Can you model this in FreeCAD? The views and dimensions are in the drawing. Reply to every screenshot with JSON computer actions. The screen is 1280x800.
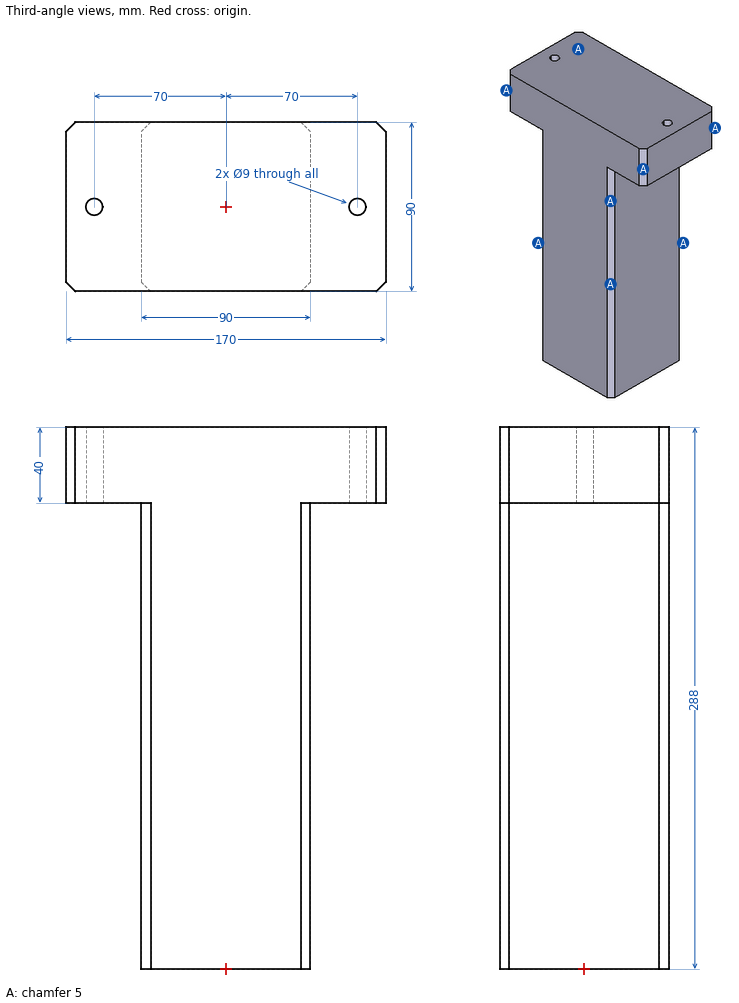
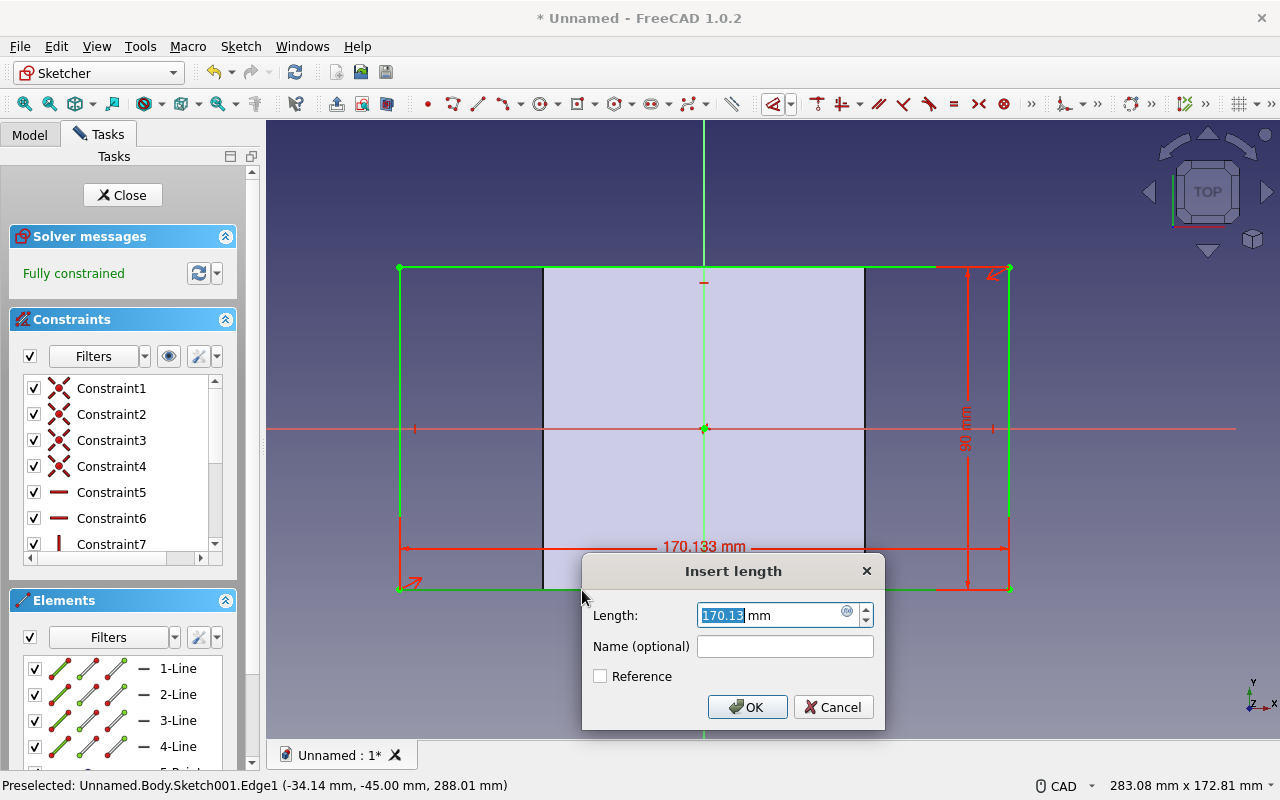
{"action": "type", "text": "170"}
{"action": "key", "text": "Return"}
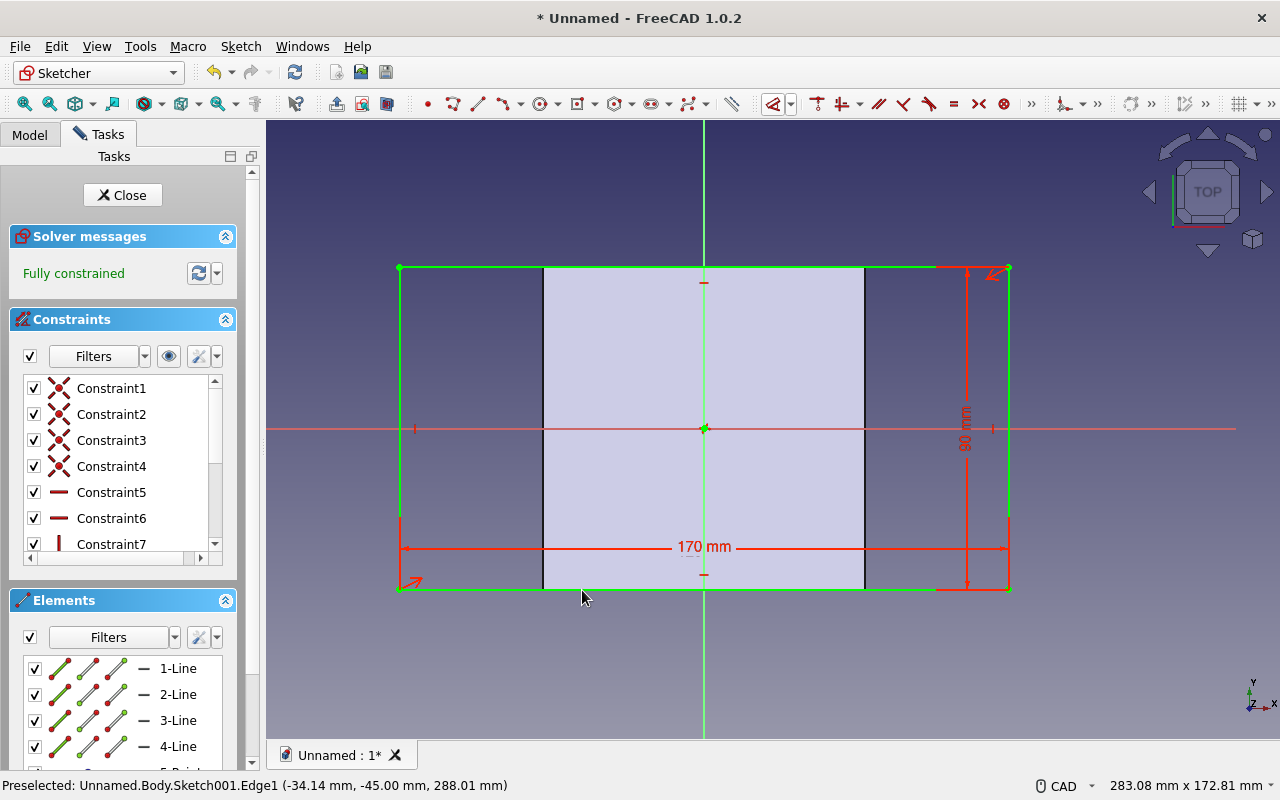
{"action": "left_click", "coordinate": [123, 195]}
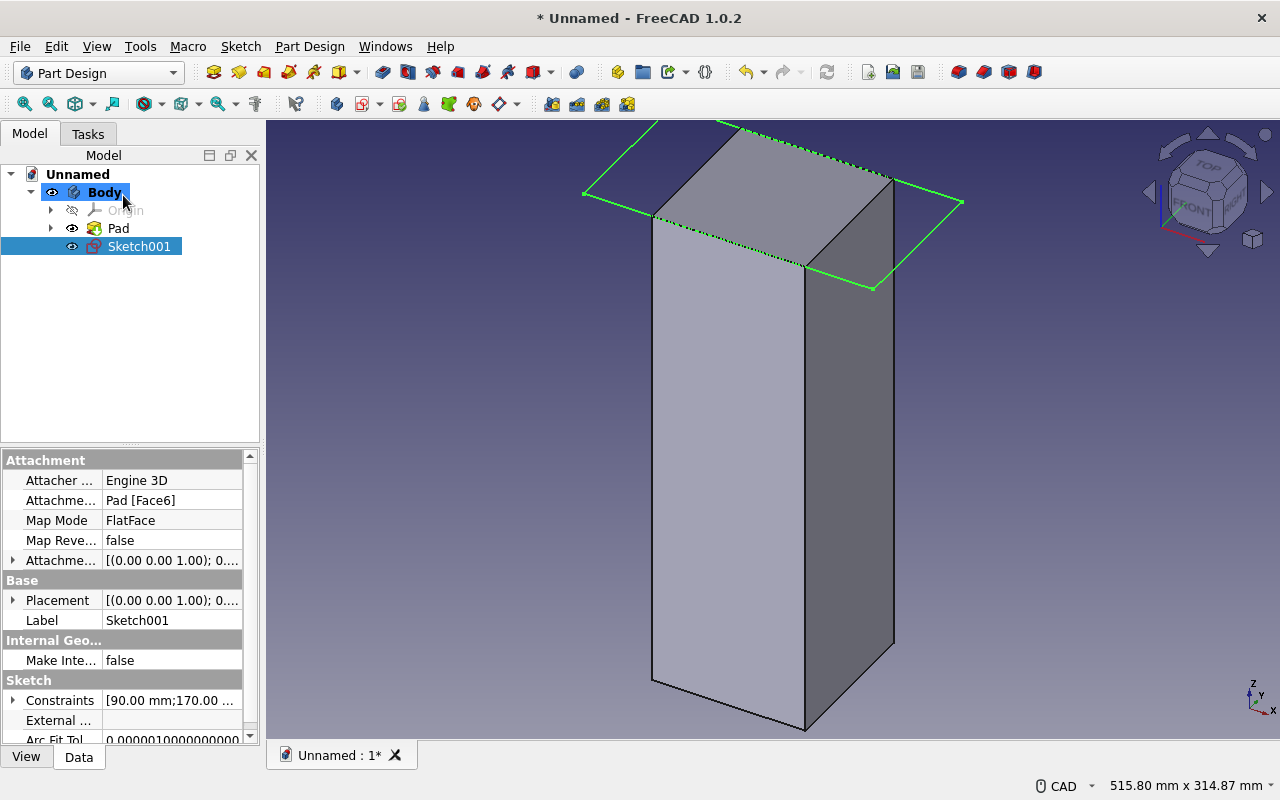
{"action": "left_click", "coordinate": [214, 72]}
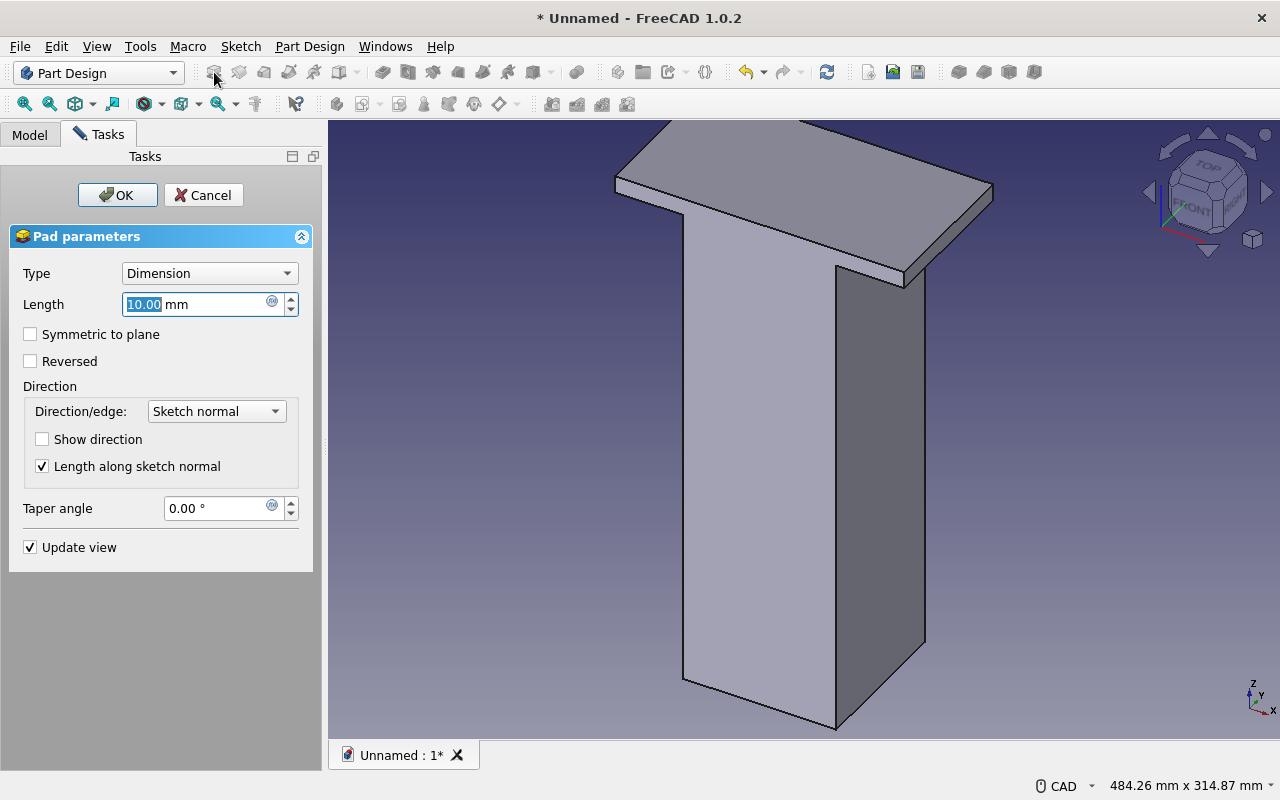
{"action": "type", "text": "40"}
{"action": "key", "text": "Tab"}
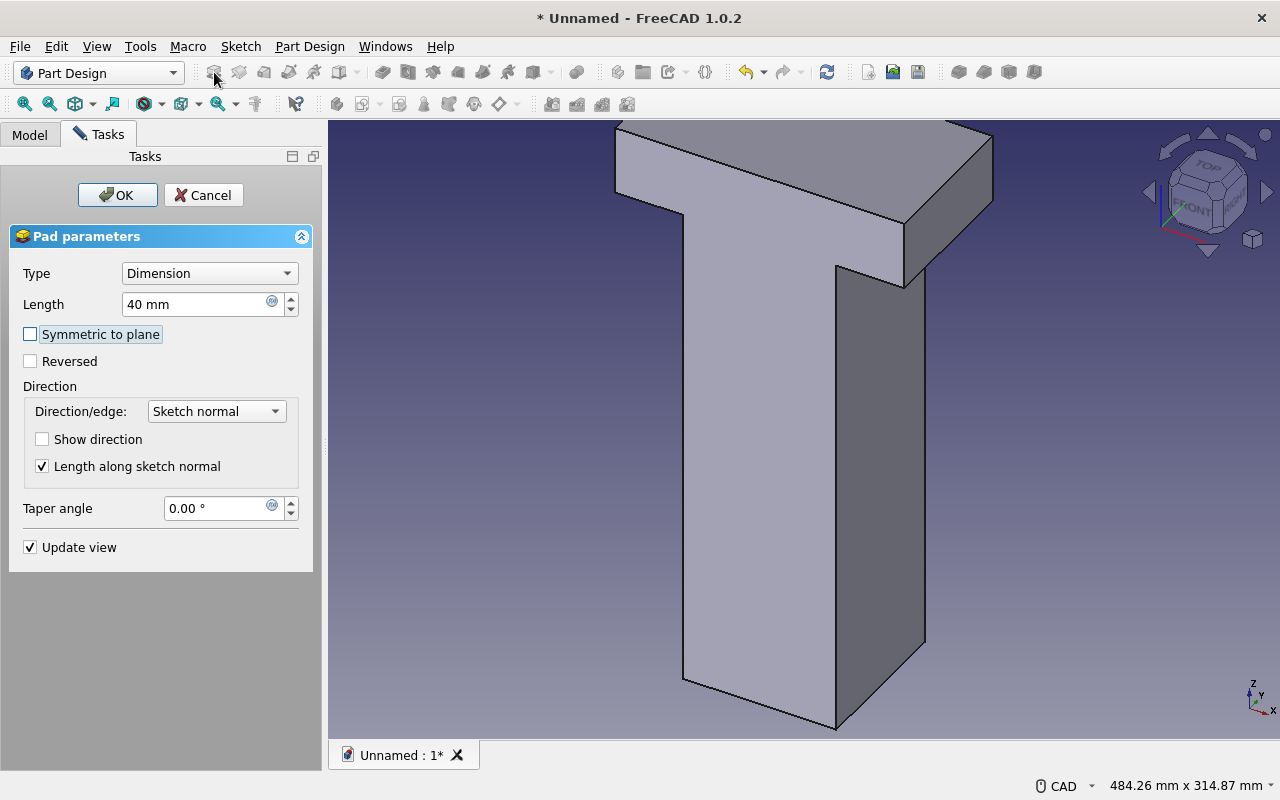
{"action": "left_click", "coordinate": [31, 361]}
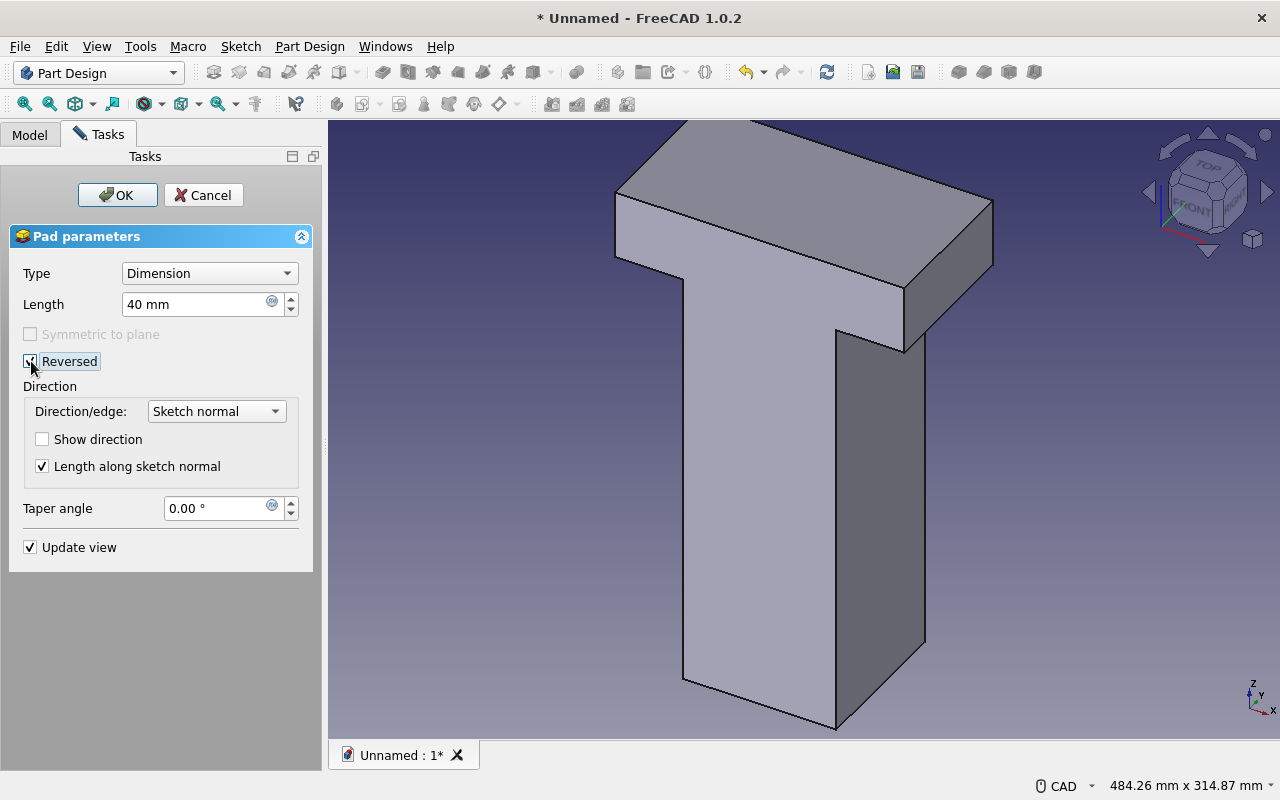
{"action": "left_click", "coordinate": [118, 195]}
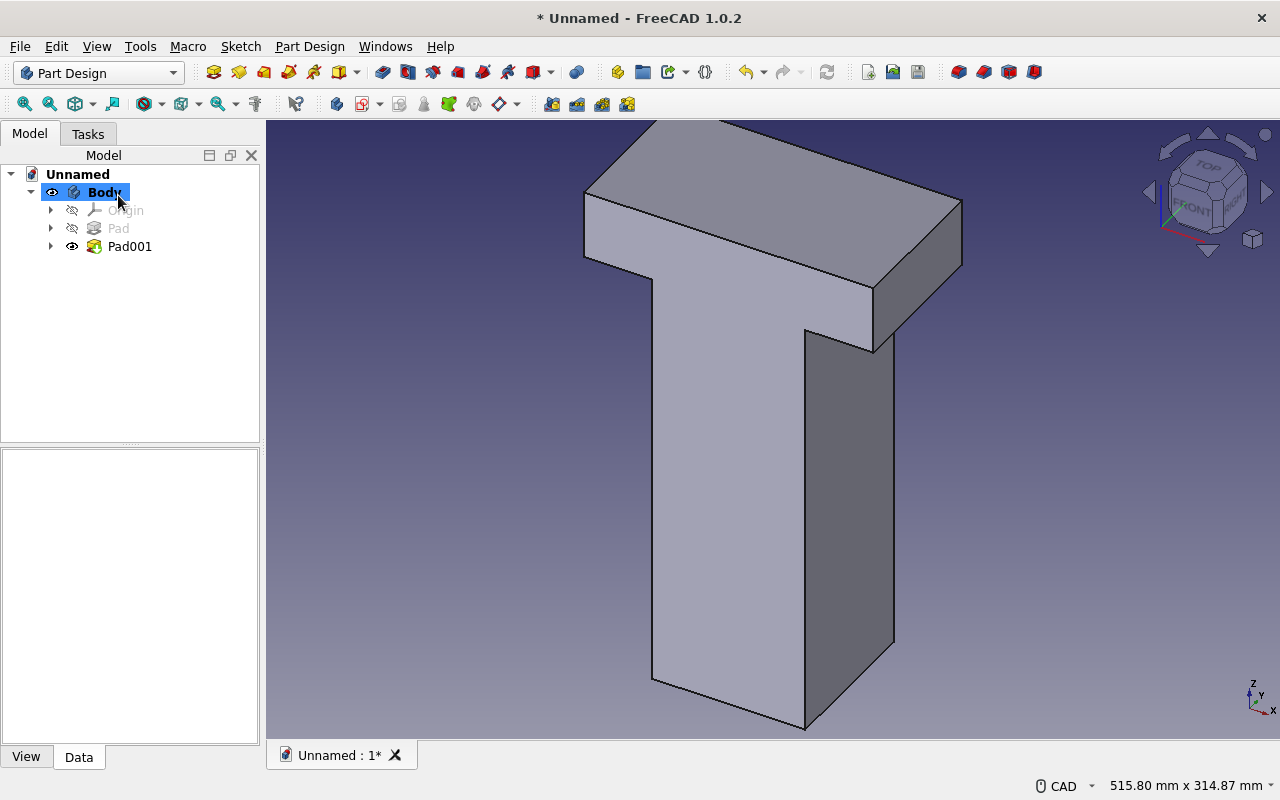
{"action": "left_click", "coordinate": [25, 104]}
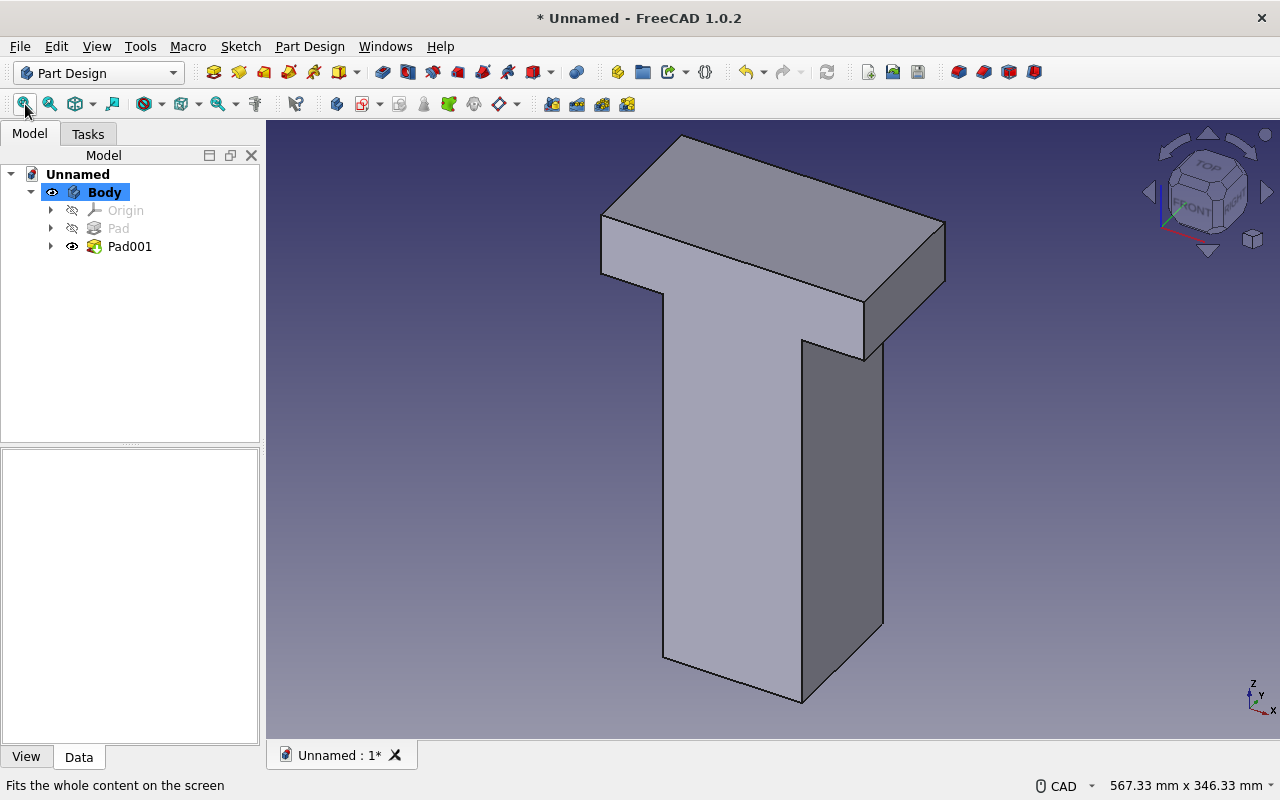
{"action": "left_click", "coordinate": [802, 521]}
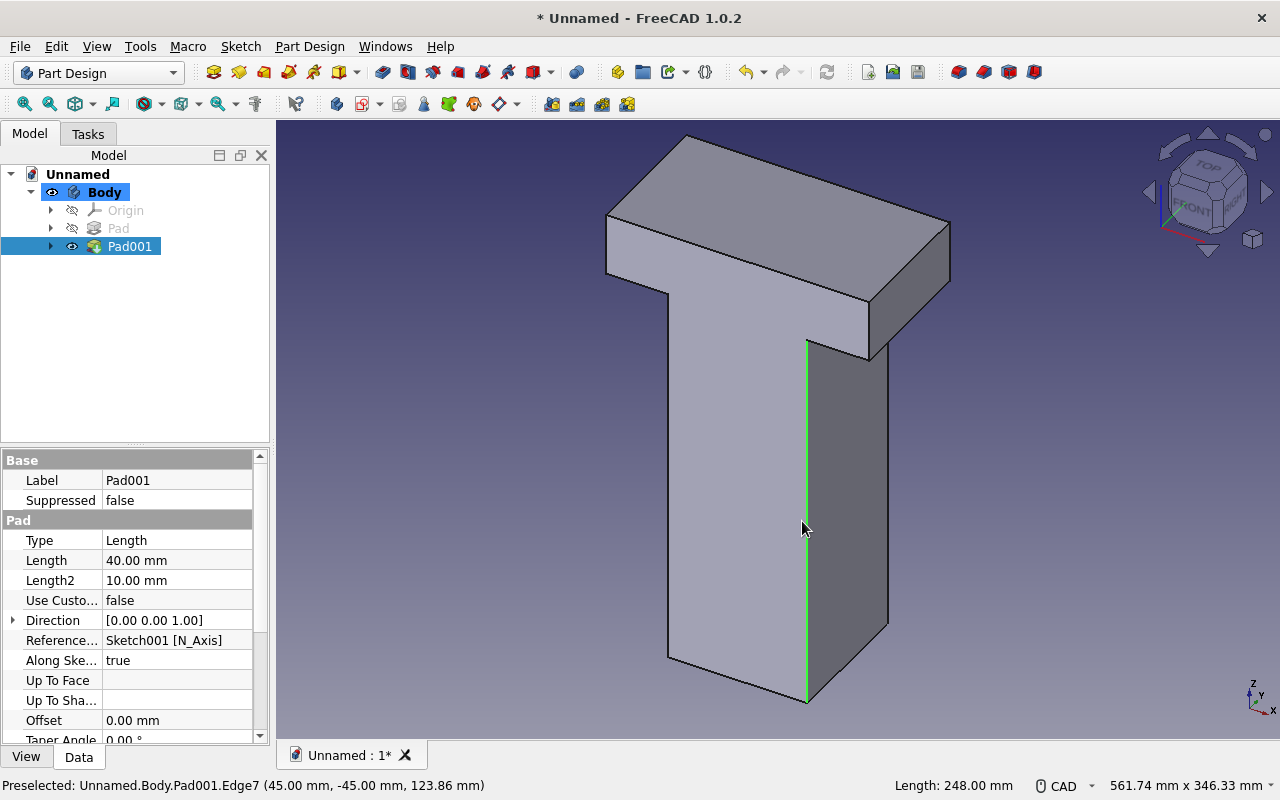
{"action": "left_click", "coordinate": [869, 330], "text": "ctrl"}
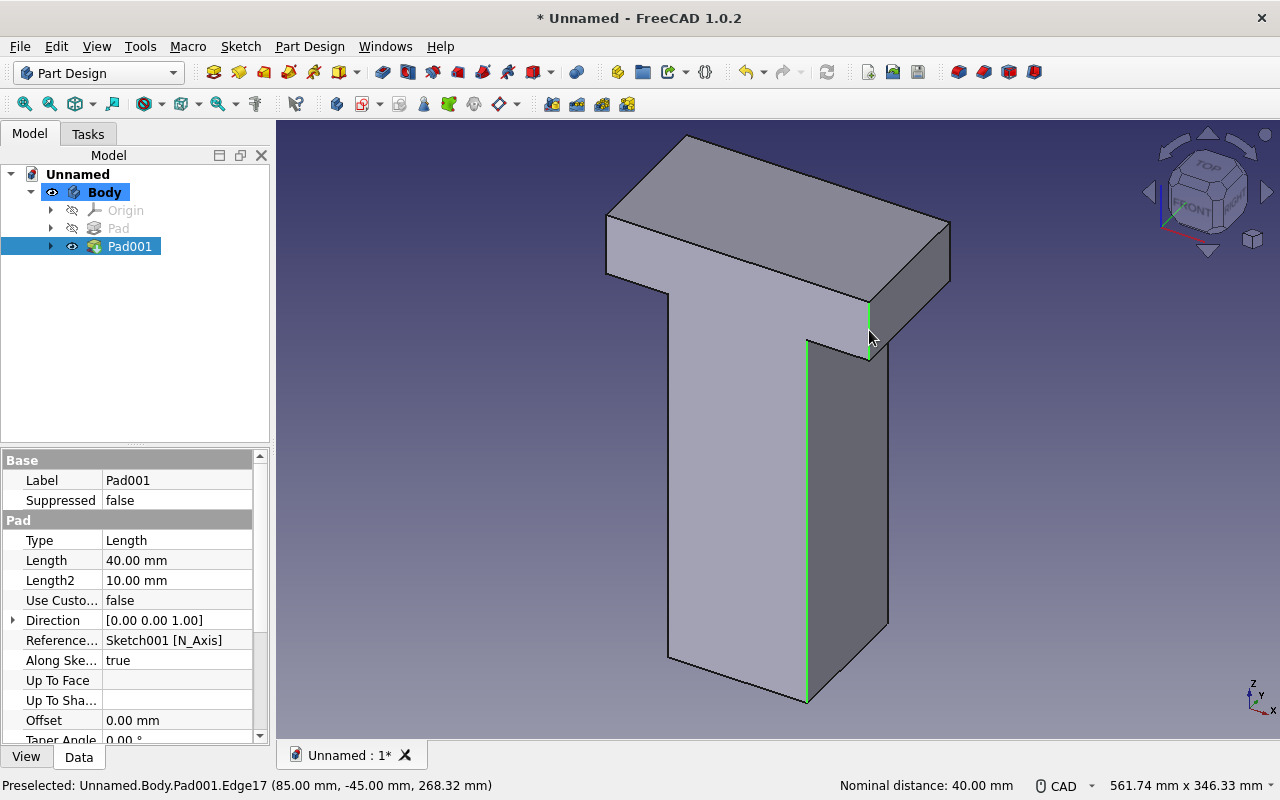
{"action": "key", "text": "0"}